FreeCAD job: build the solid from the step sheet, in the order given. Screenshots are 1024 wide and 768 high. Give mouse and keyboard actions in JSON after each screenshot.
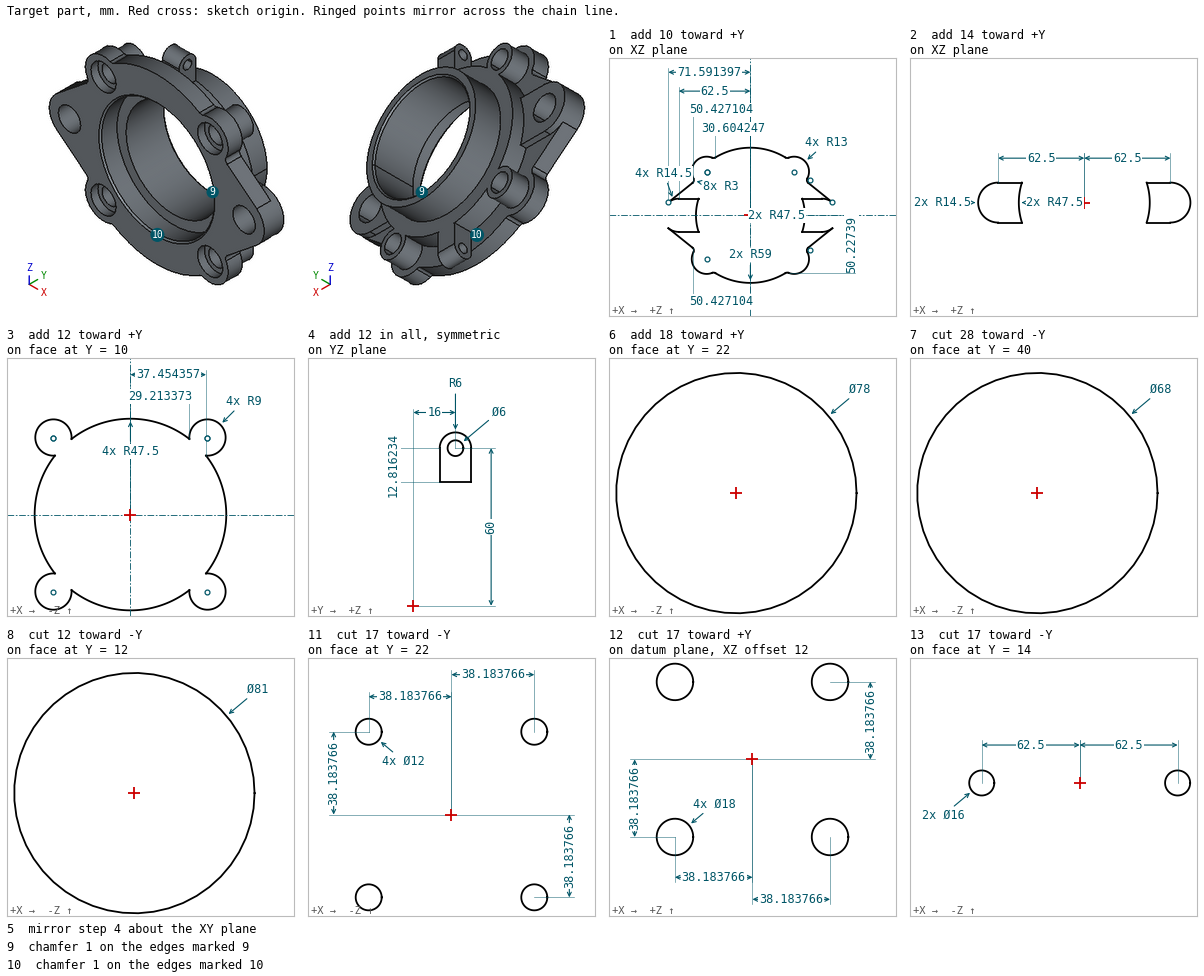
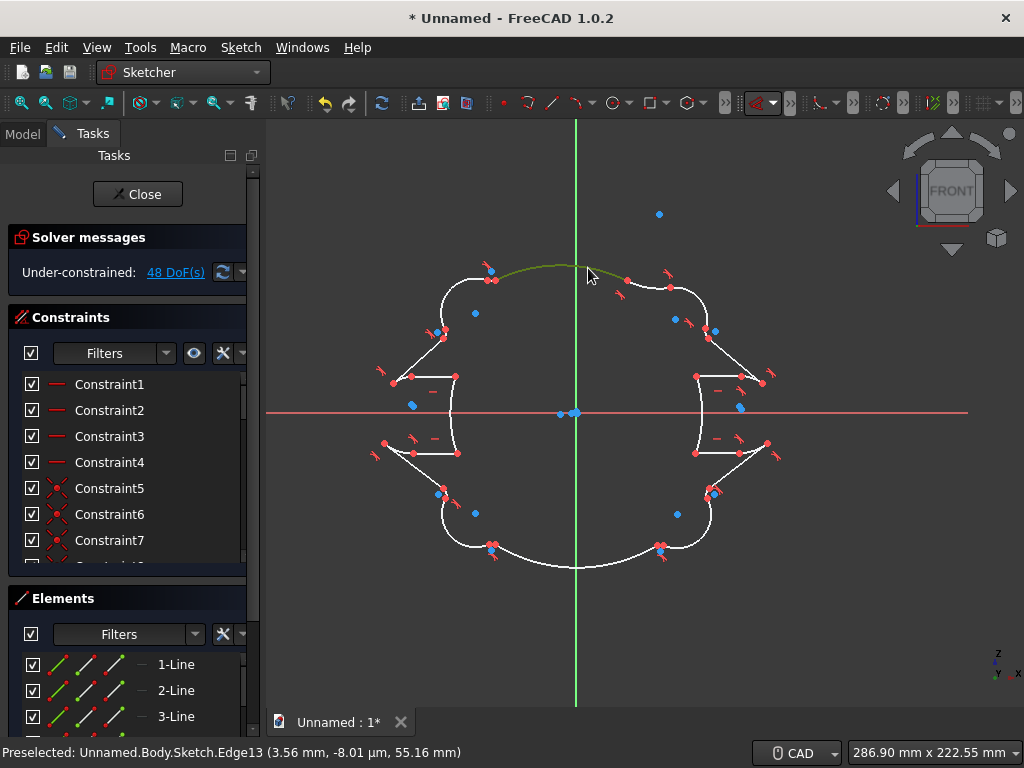
{"action": "left_click", "coordinate": [701, 430]}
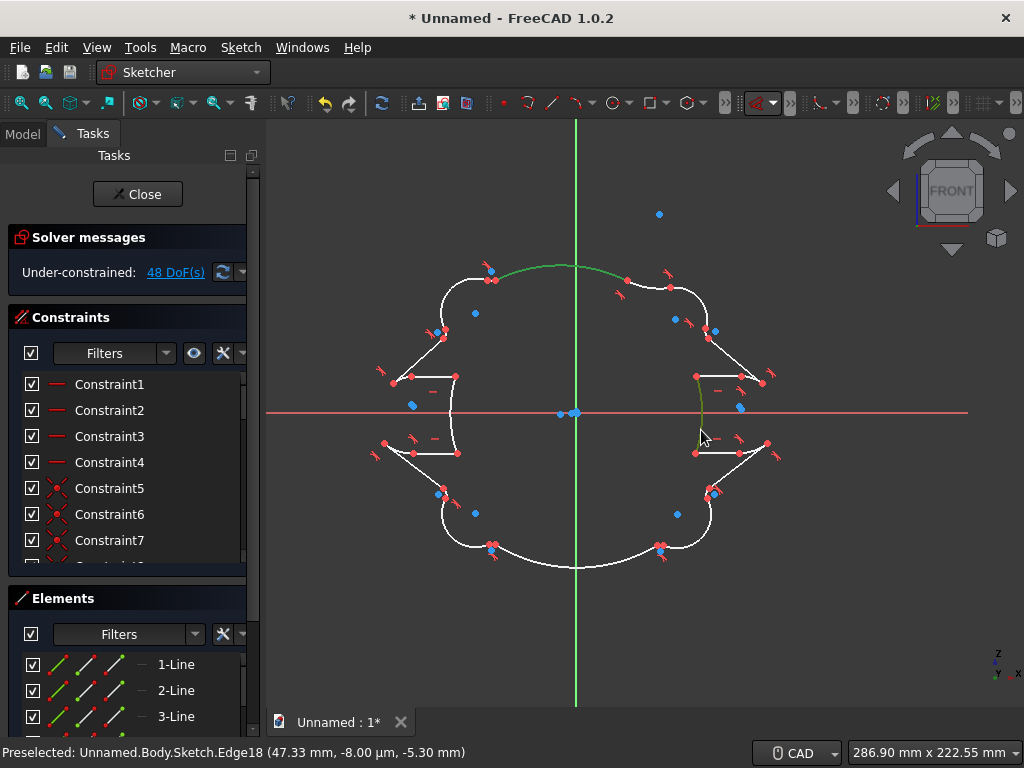
{"action": "key", "text": "c"}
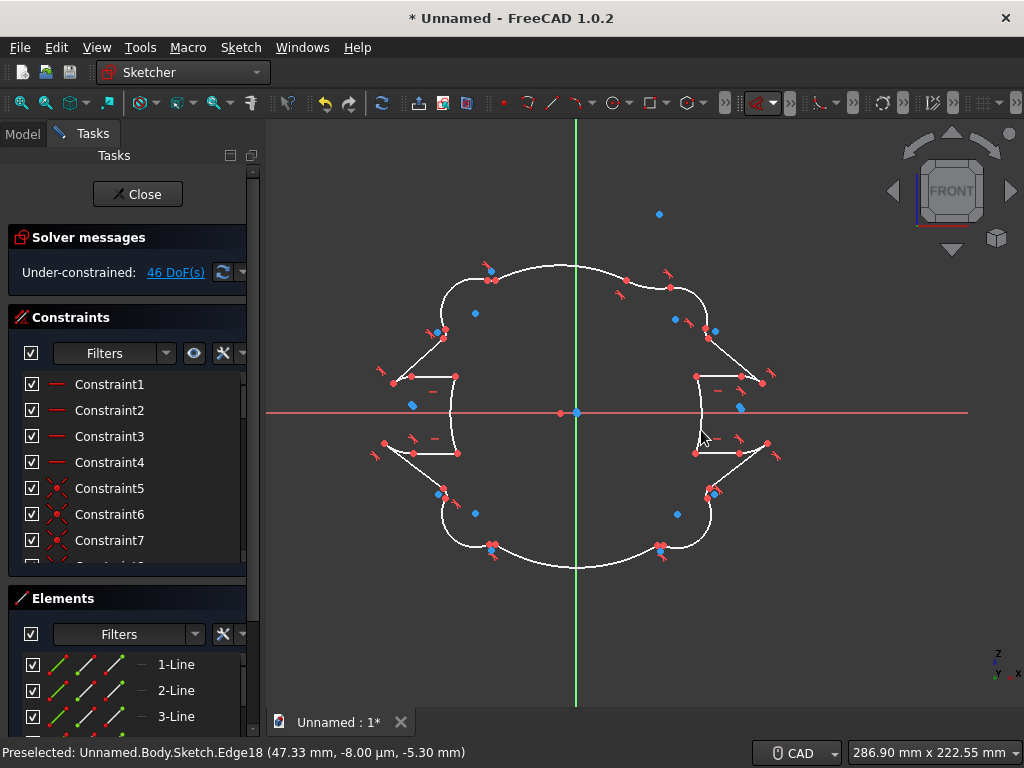
{"action": "scroll", "coordinate": [746, 377], "scroll_direction": "up", "scroll_amount": 6}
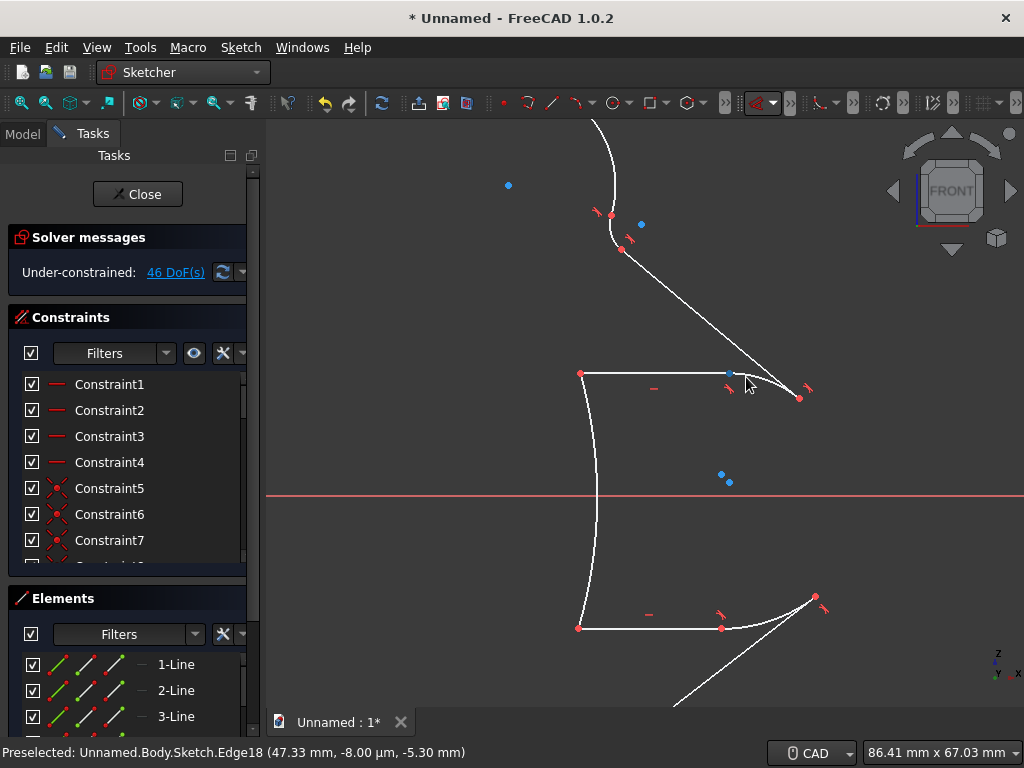
{"action": "left_click", "coordinate": [744, 374]}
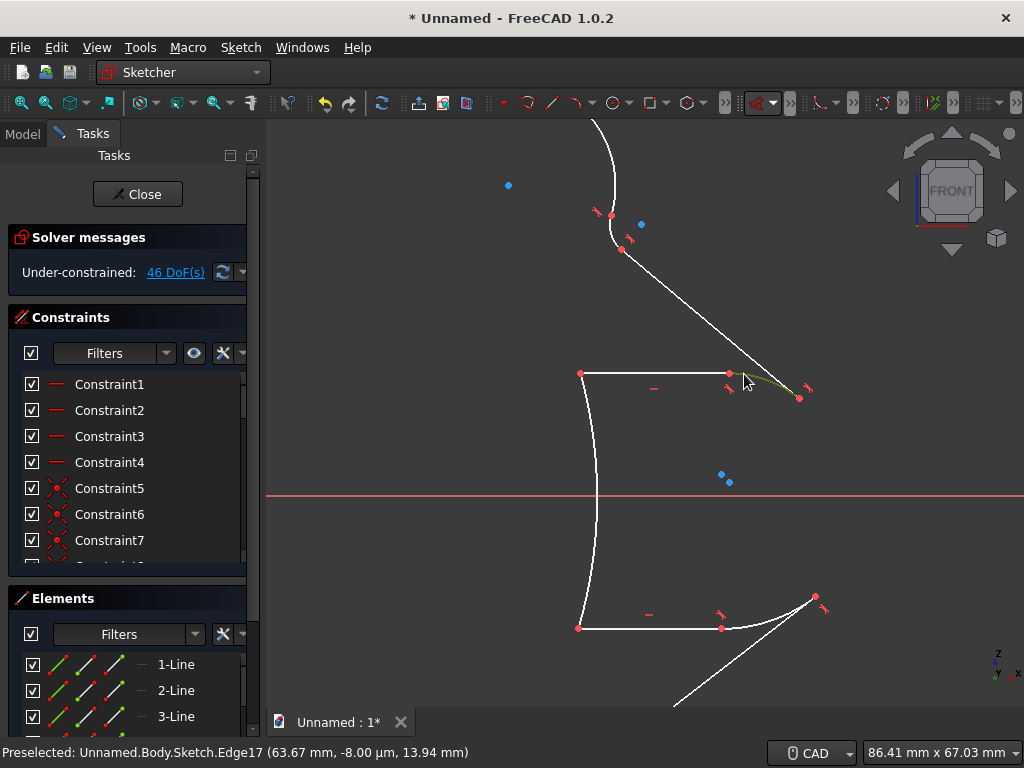
{"action": "left_click", "coordinate": [752, 626]}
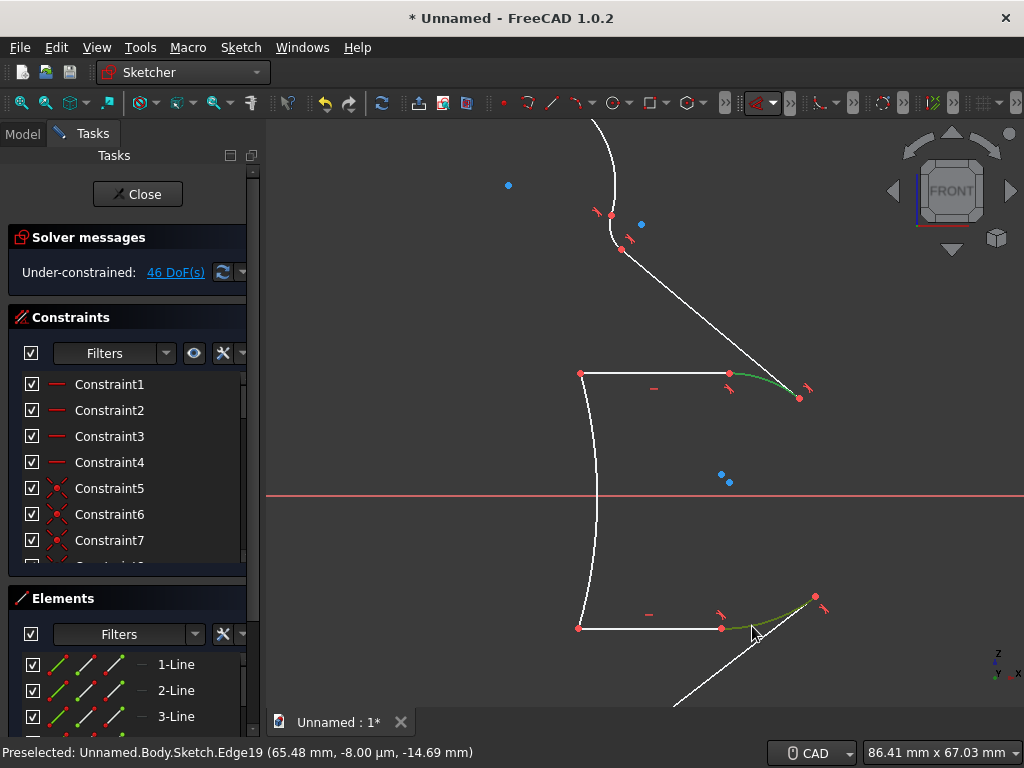
{"action": "key", "text": "c"}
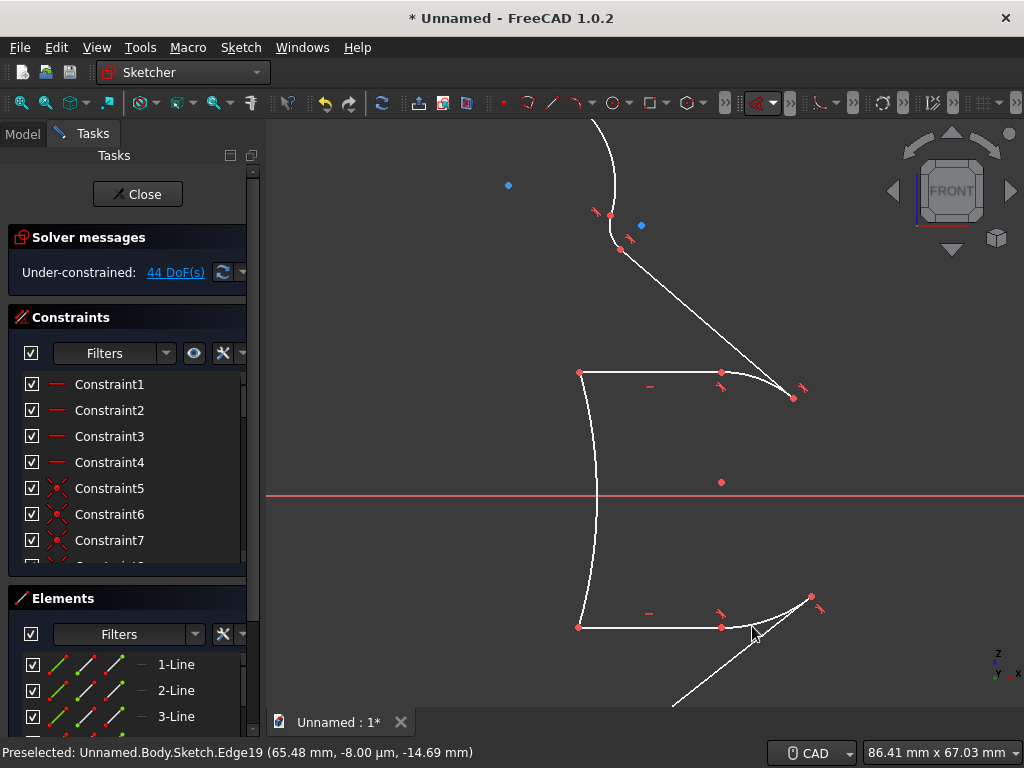
{"action": "scroll", "coordinate": [747, 377], "scroll_direction": "down", "scroll_amount": 6}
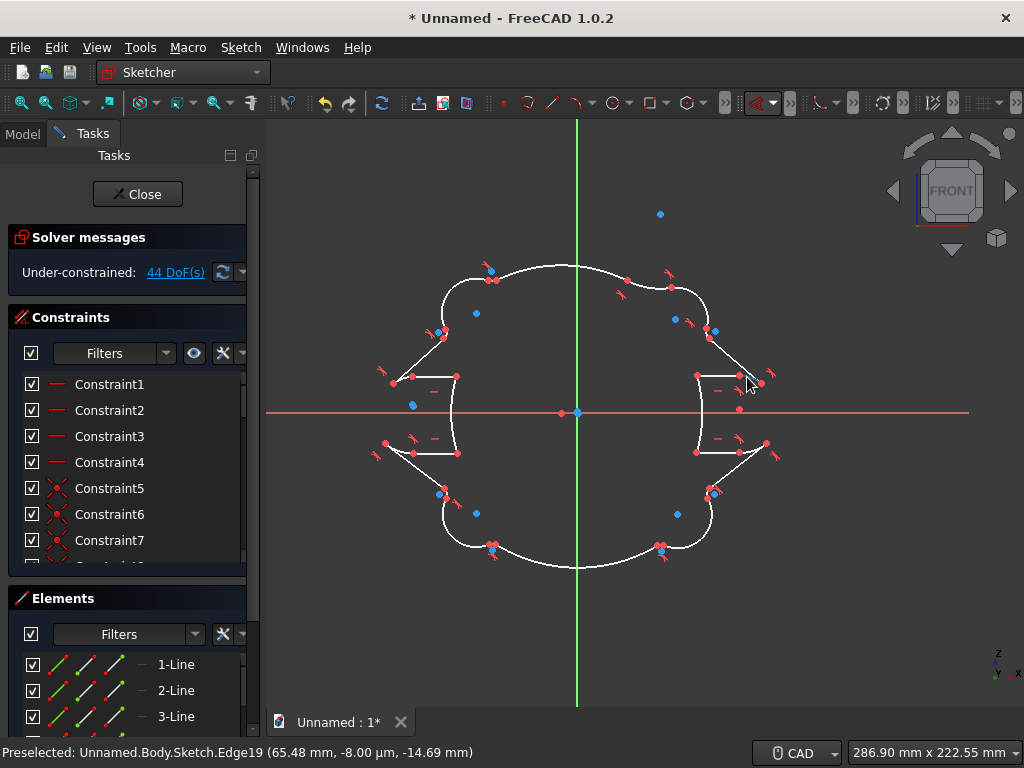
{"action": "left_click", "coordinate": [589, 268]}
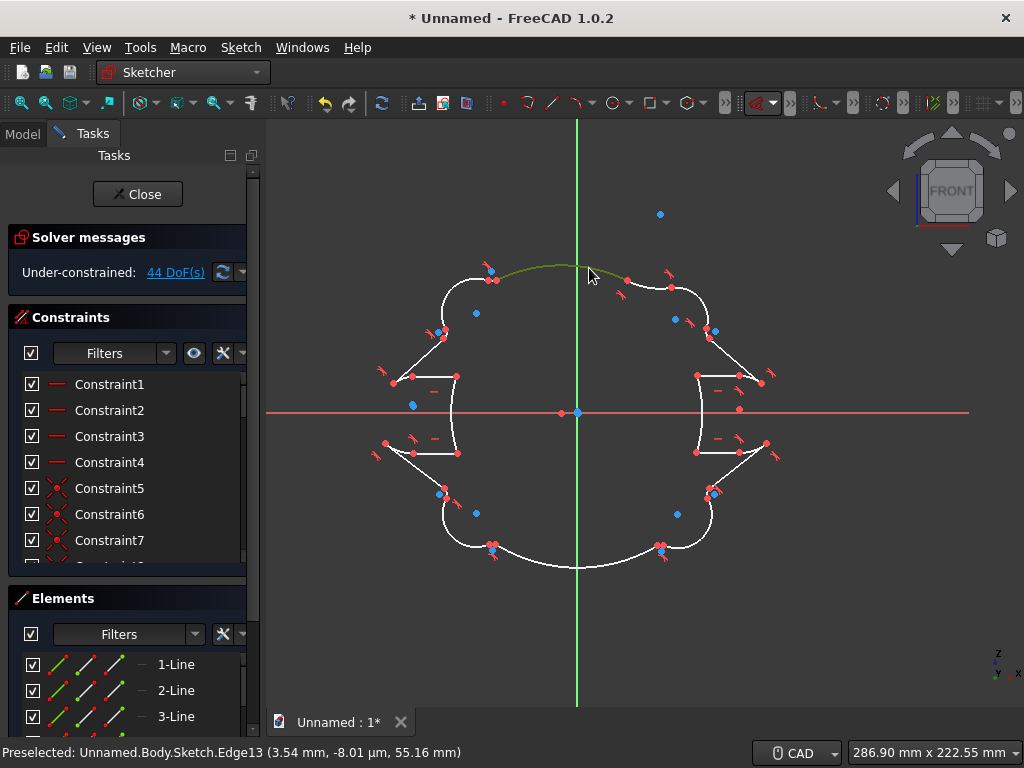
{"action": "left_click", "coordinate": [543, 564]}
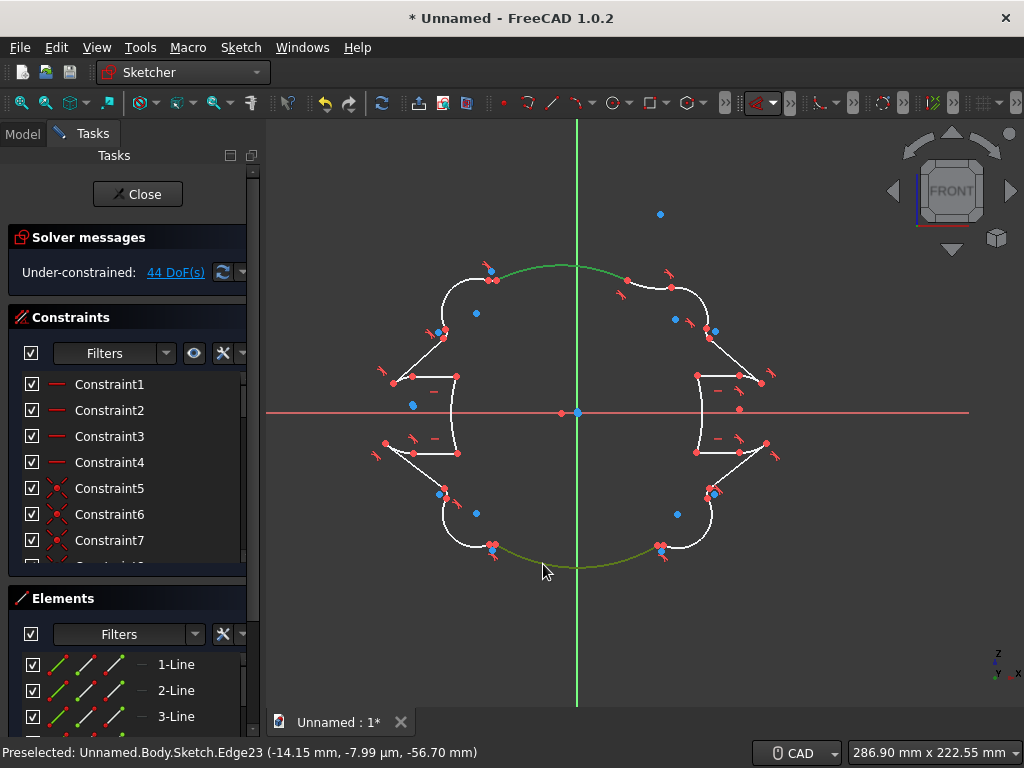
{"action": "key", "text": "c"}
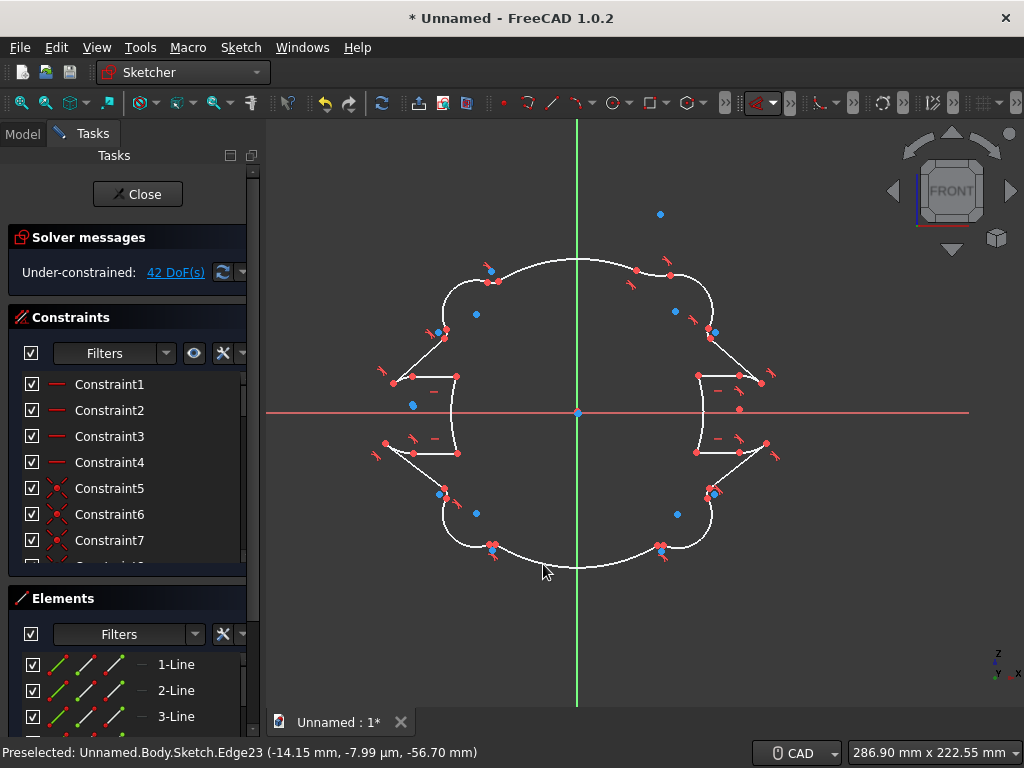
{"action": "scroll", "coordinate": [408, 377], "scroll_direction": "up", "scroll_amount": 7}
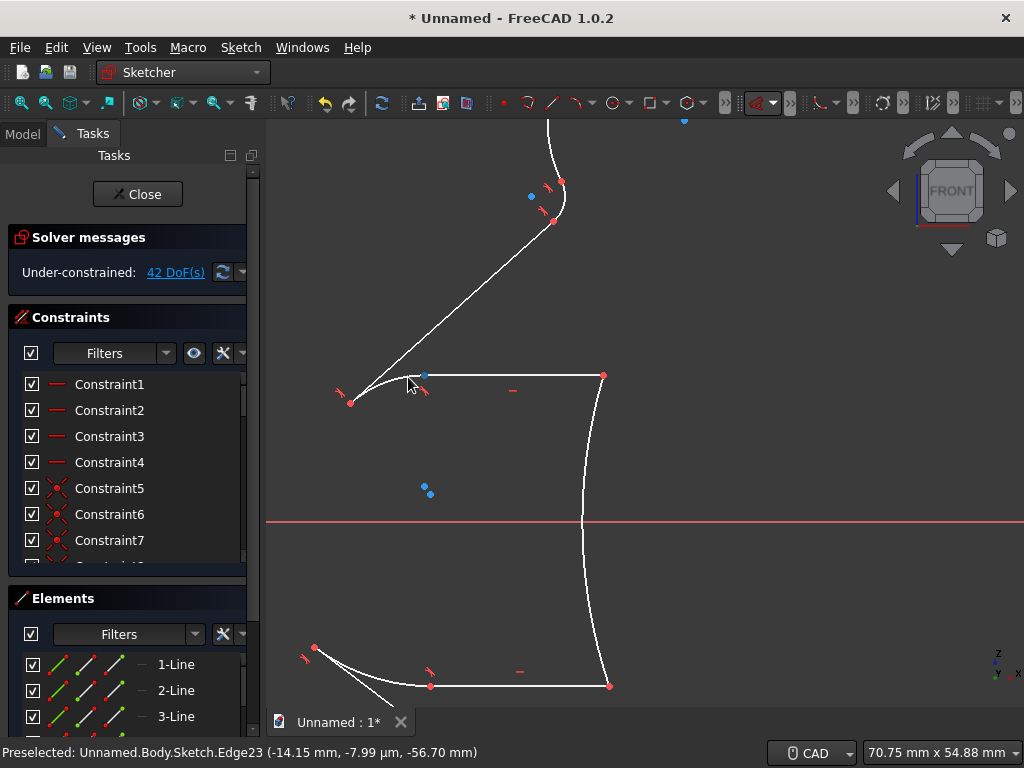
{"action": "left_click", "coordinate": [408, 377]}